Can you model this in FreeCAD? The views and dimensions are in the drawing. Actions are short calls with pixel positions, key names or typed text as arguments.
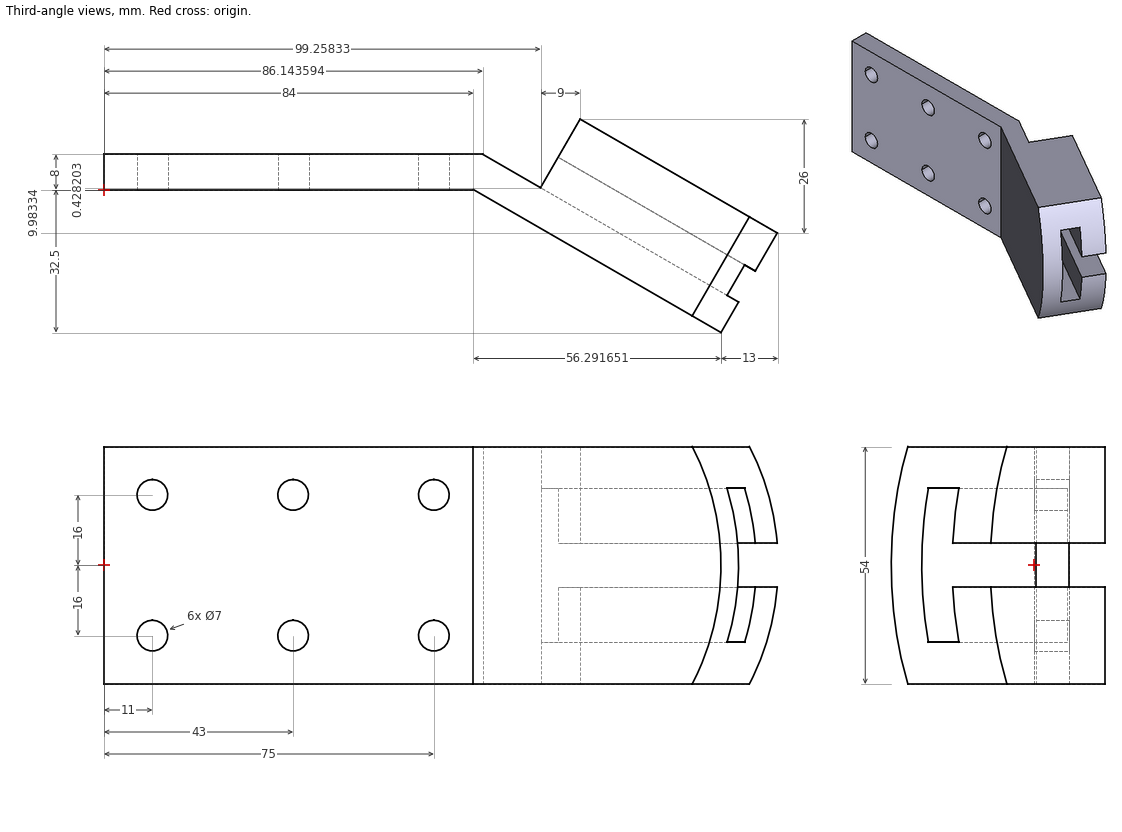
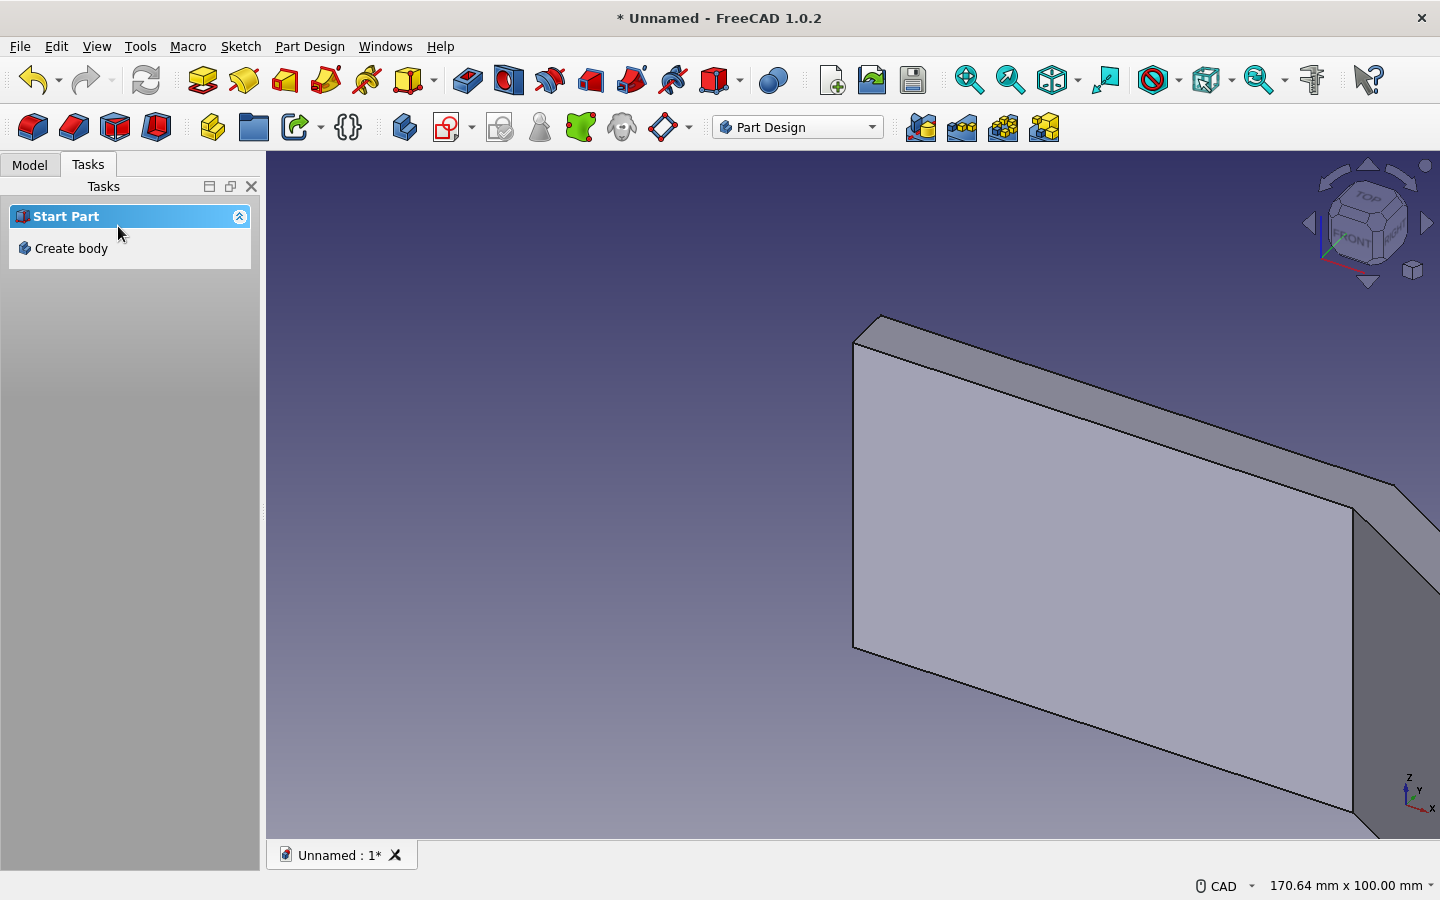
key(v)
key(f)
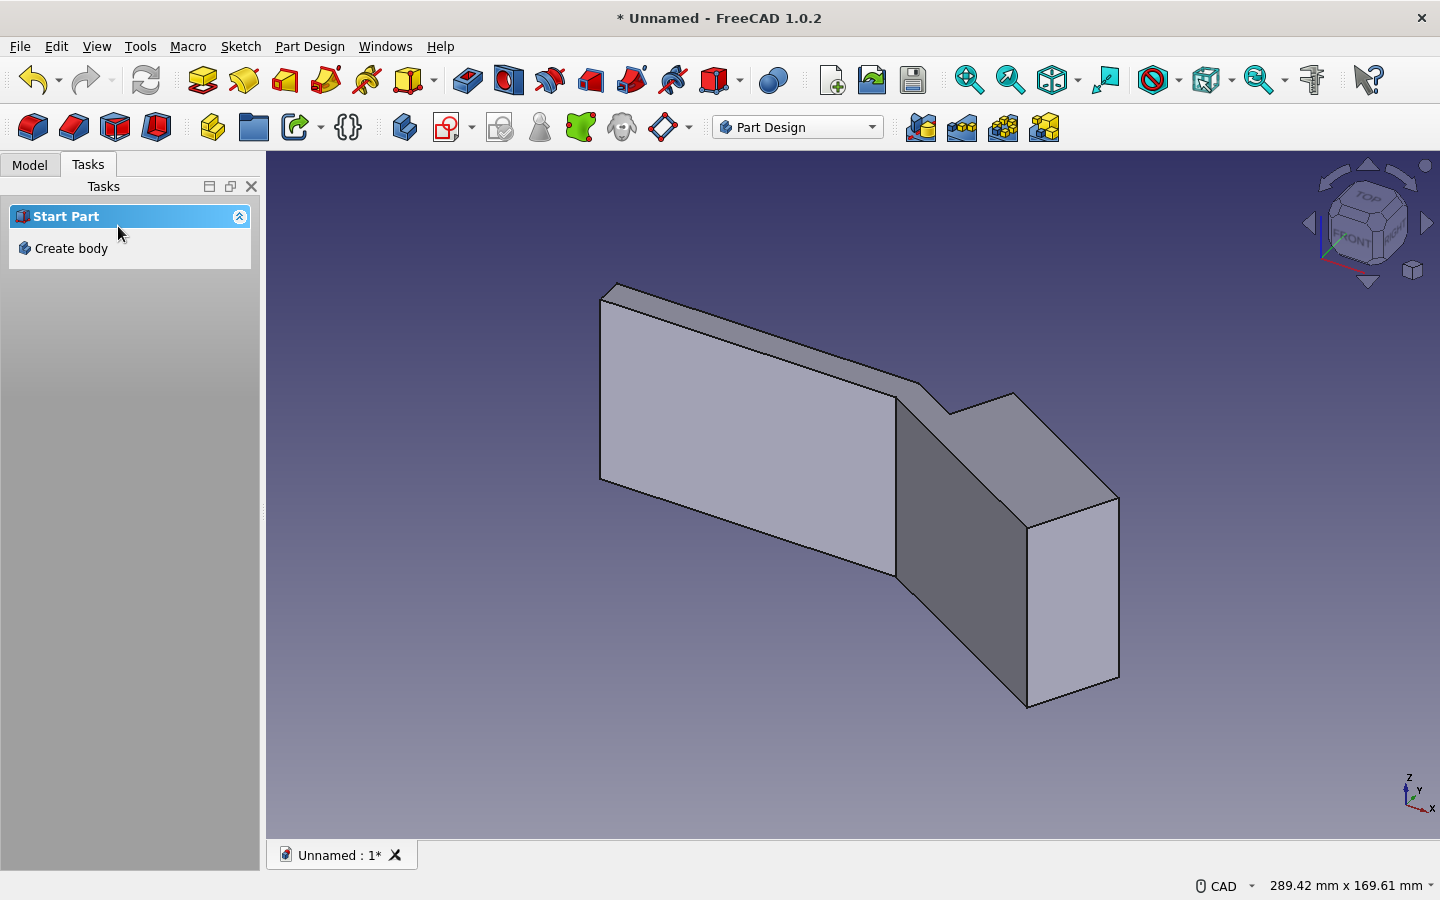
click(1073, 576)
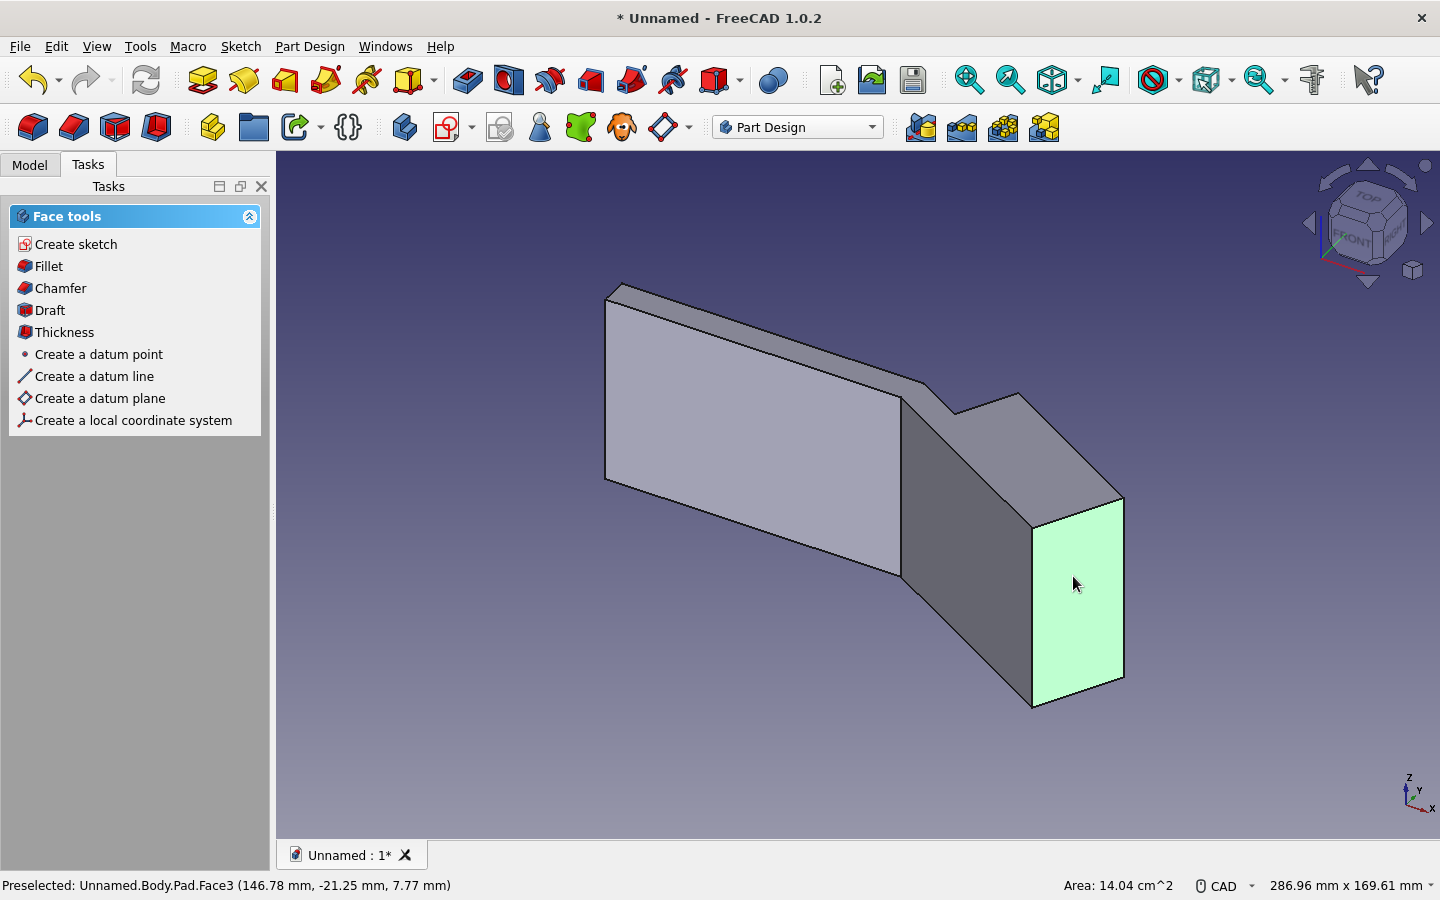
click(446, 128)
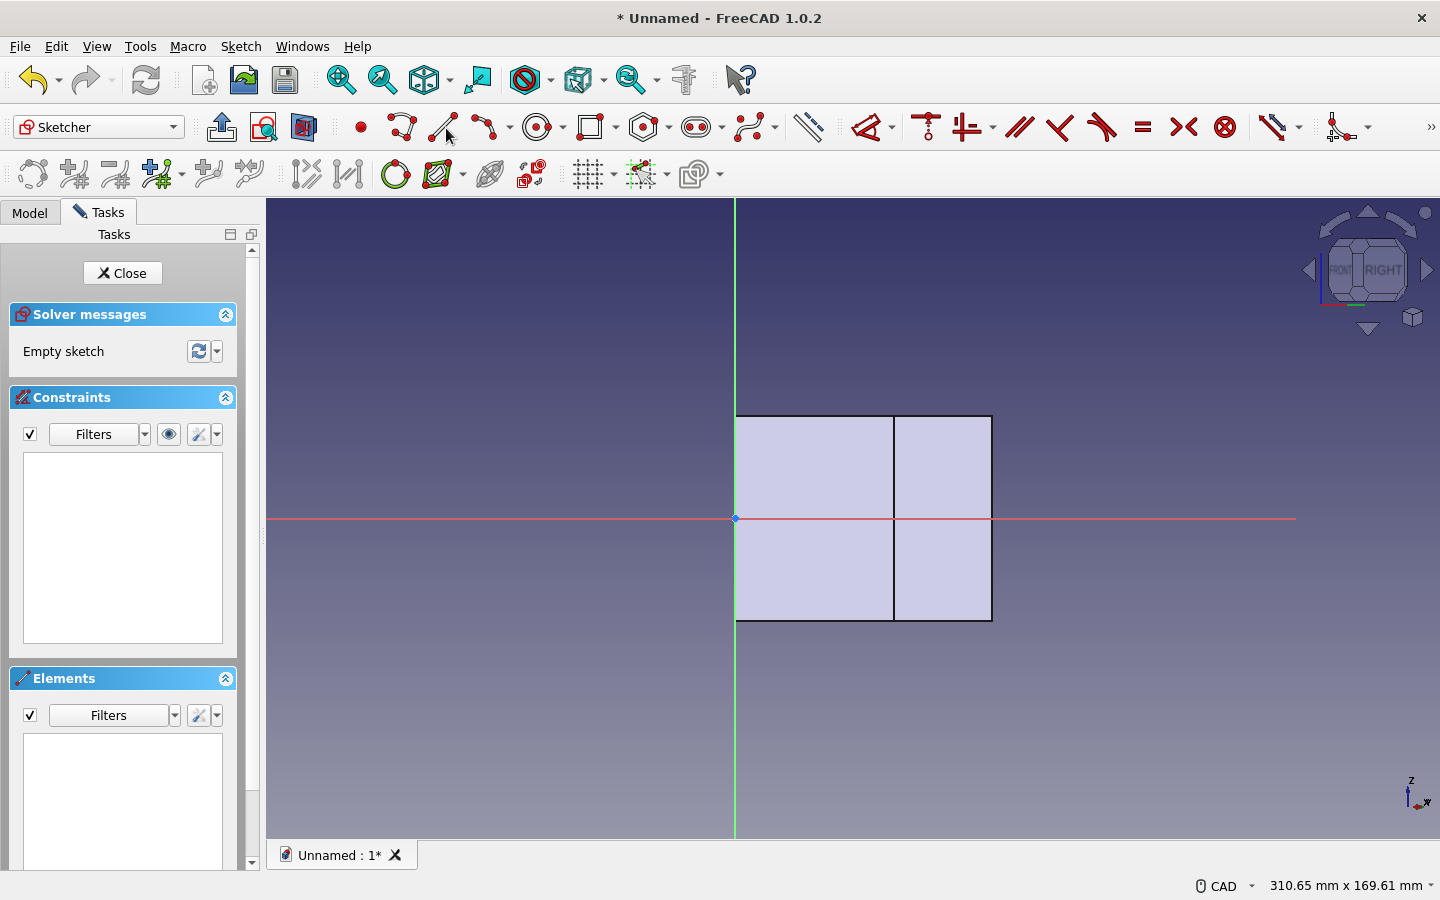
key(q)
key(s)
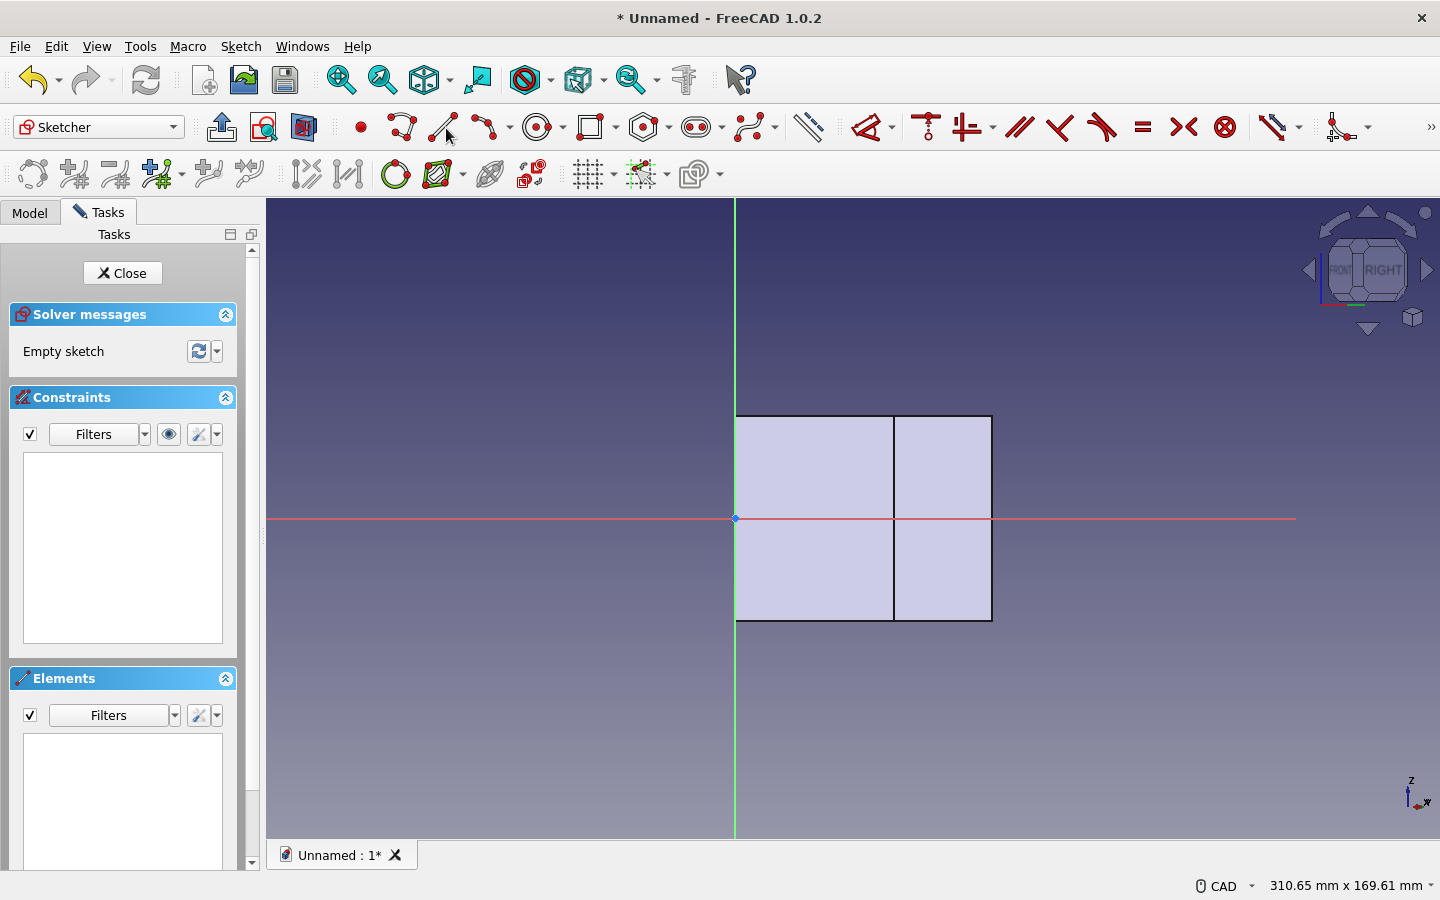
scroll(910, 518, up, 5)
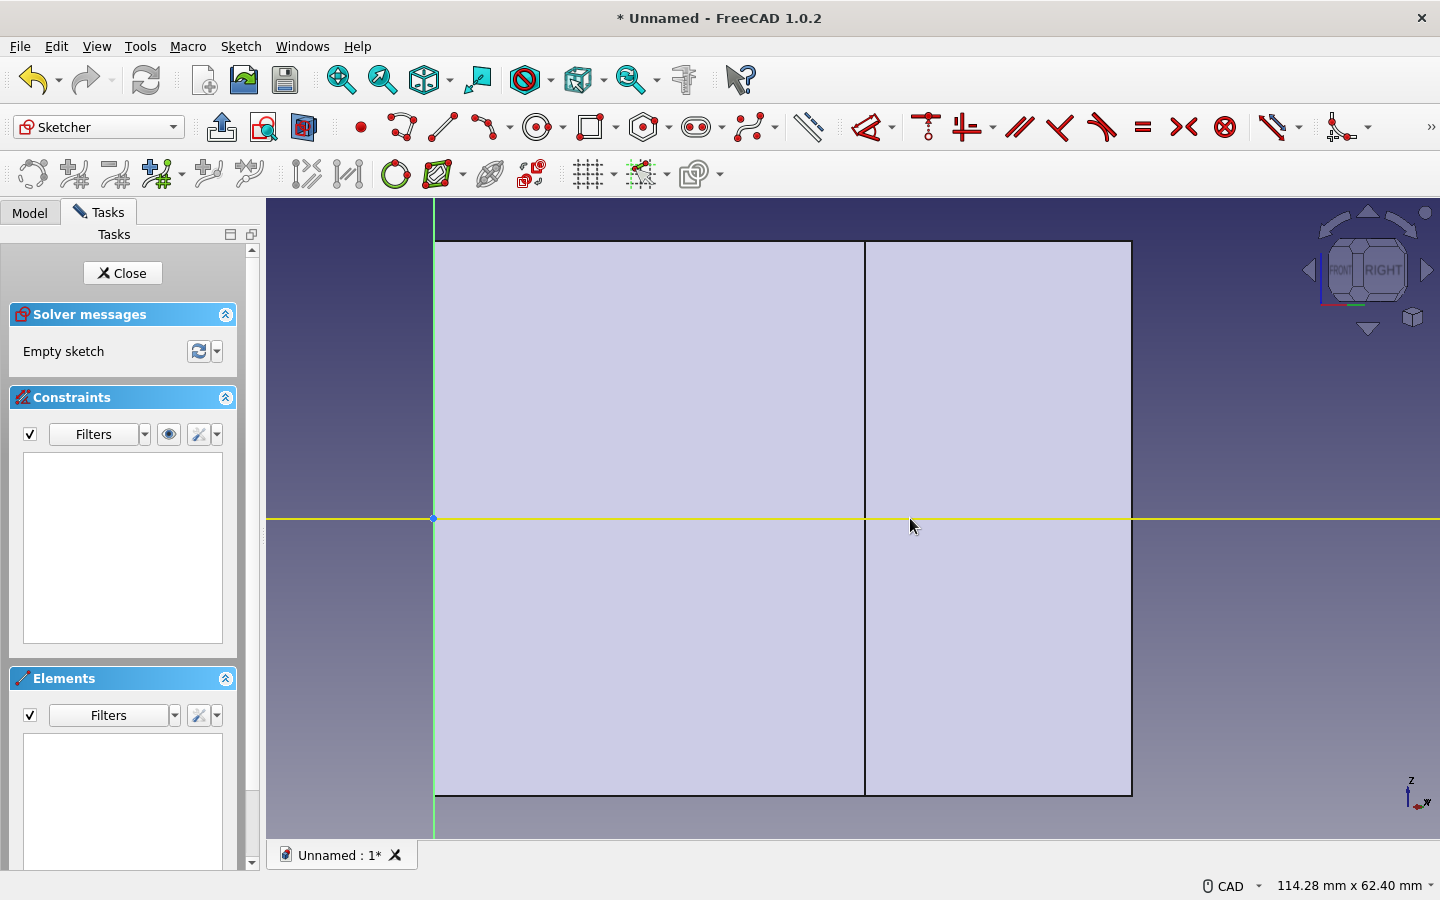
key(g)
key(m)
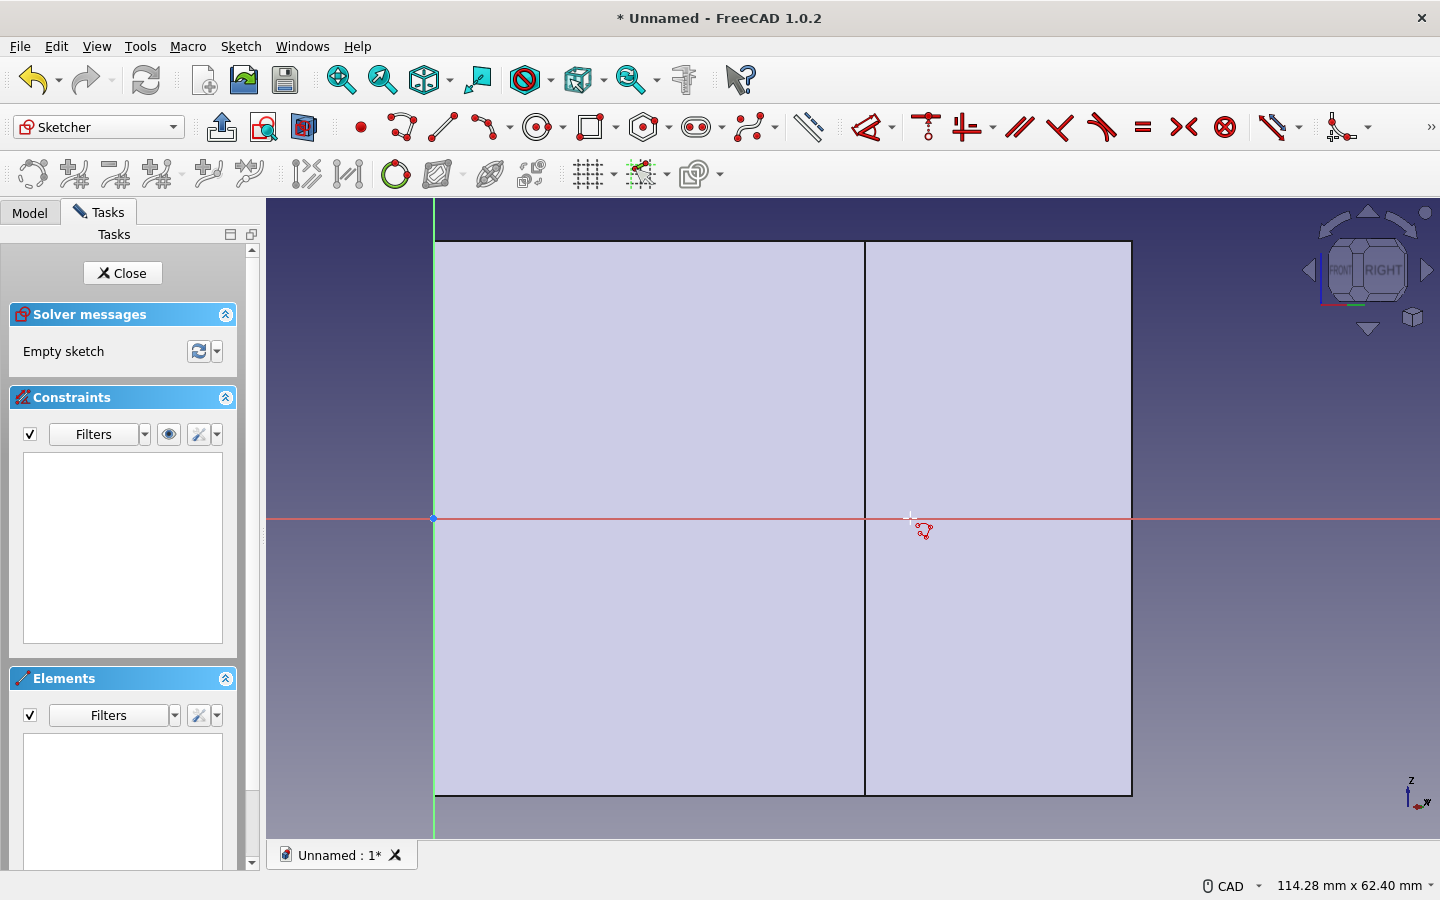
click(947, 339)
click(947, 698)
click(1030, 698)
click(1030, 570)
click(1132, 570)
click(1132, 467)
click(1030, 467)
click(1030, 339)
click(947, 340)
key(Escape)
key(Escape)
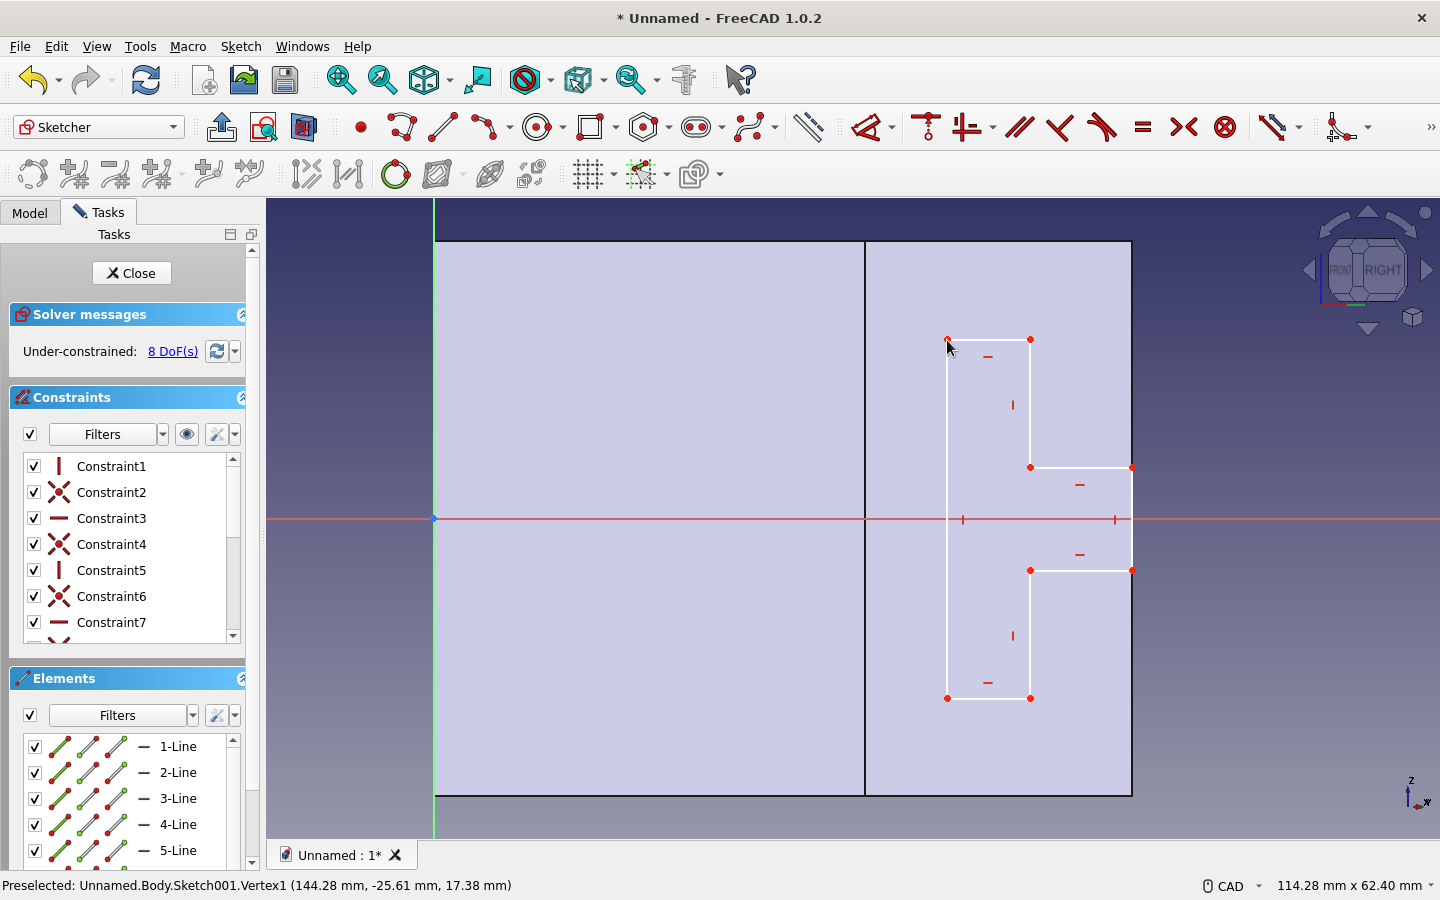
click(1030, 571)